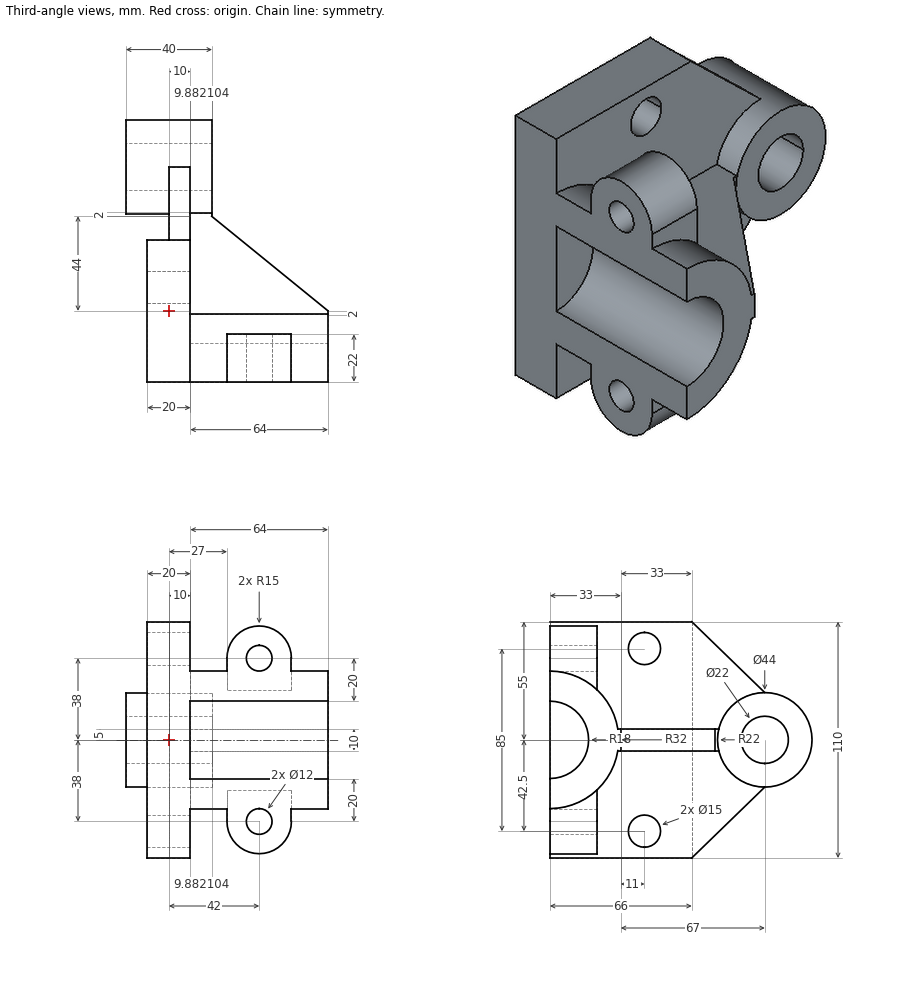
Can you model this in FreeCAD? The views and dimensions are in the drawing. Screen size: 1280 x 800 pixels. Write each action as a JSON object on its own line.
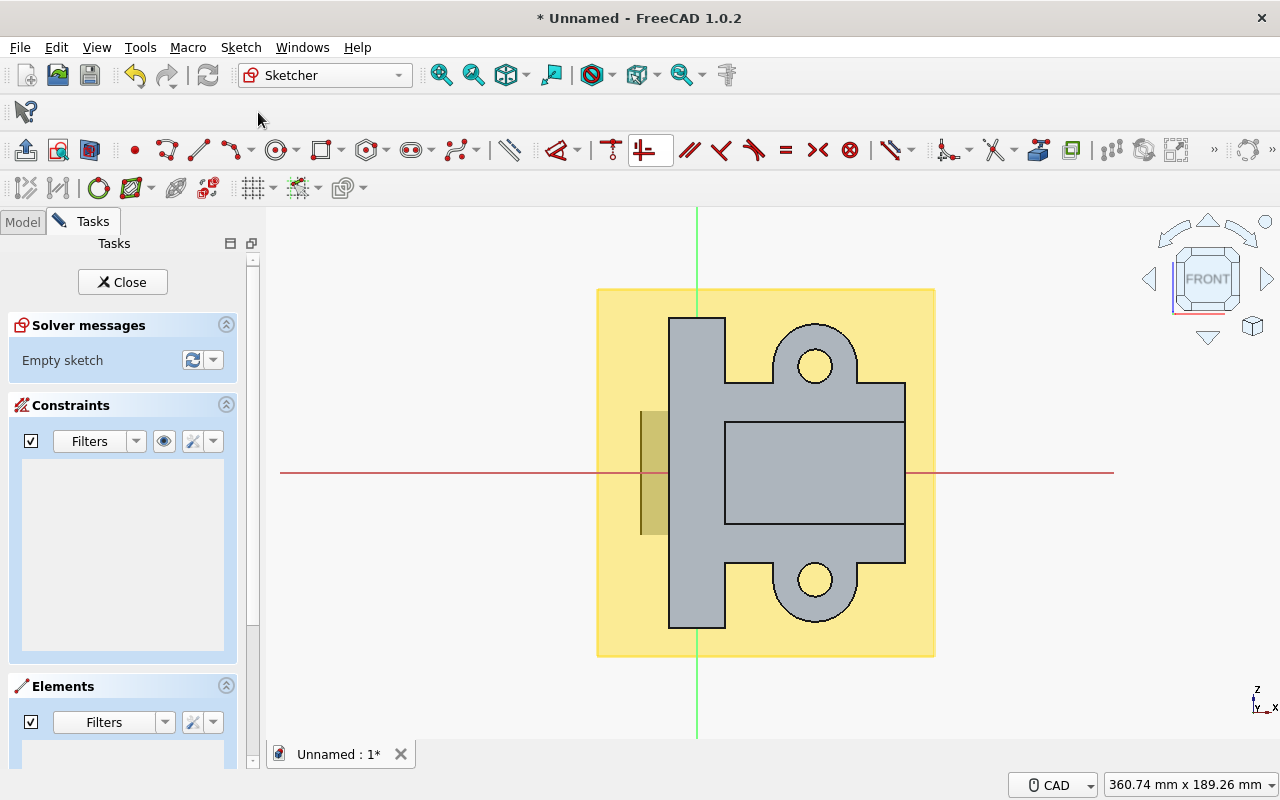
{"action": "left_click", "coordinate": [90, 150]}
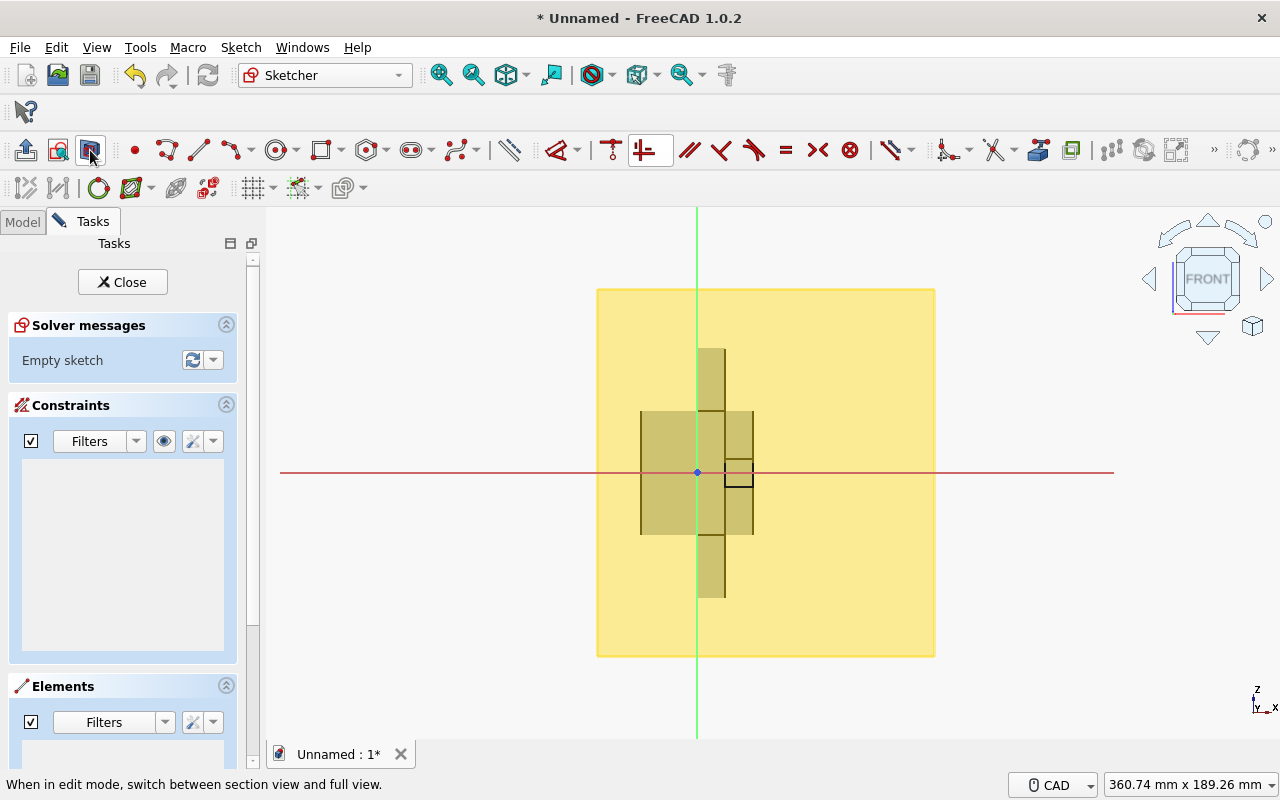
{"action": "scroll", "coordinate": [727, 473], "scroll_direction": "up", "scroll_amount": 12}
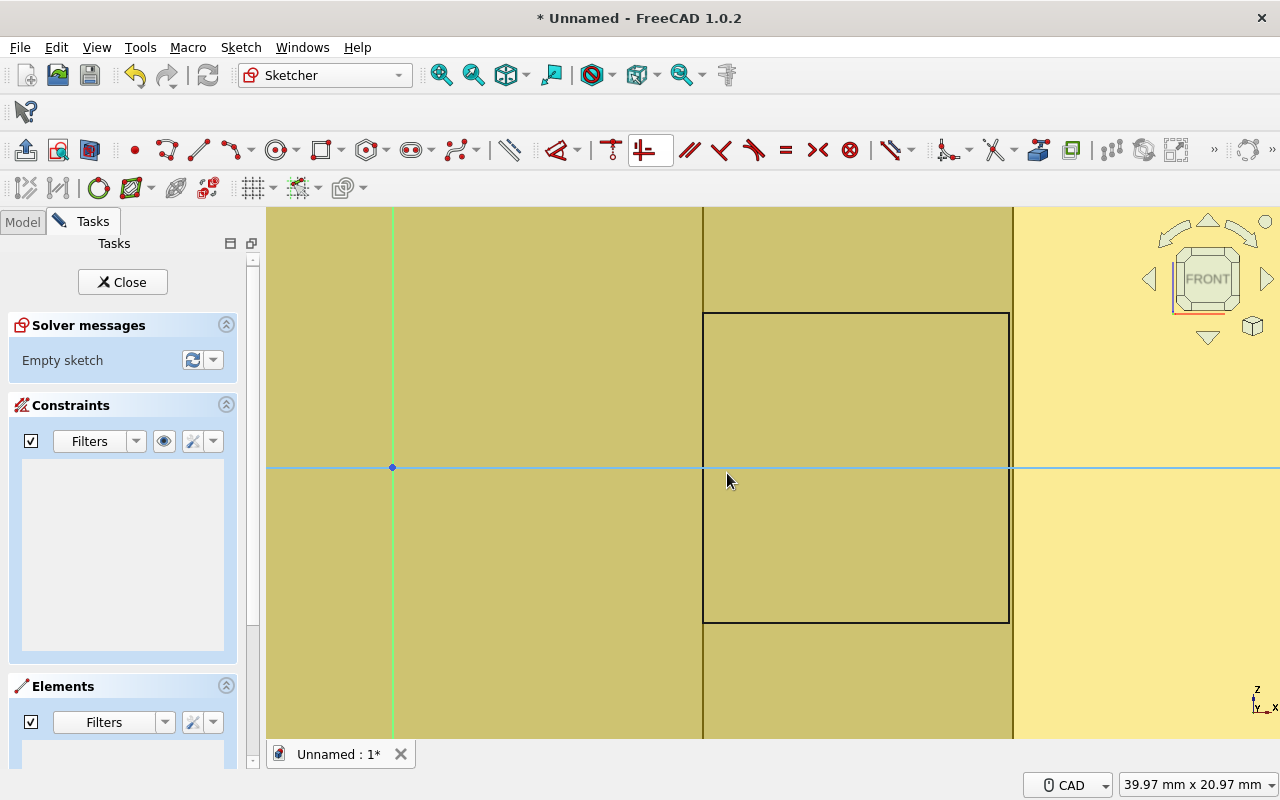
{"action": "left_click", "coordinate": [322, 150]}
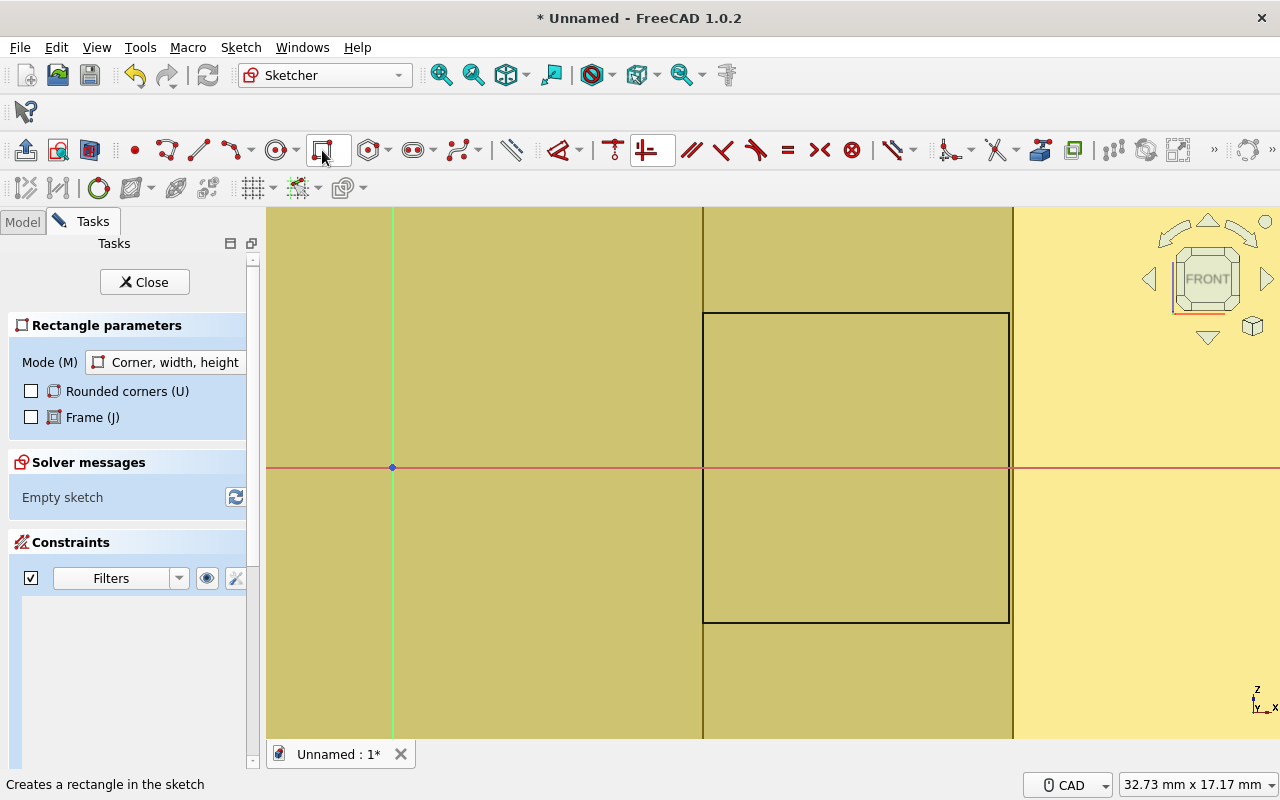
{"action": "left_click", "coordinate": [703, 313]}
{"action": "left_click", "coordinate": [1009, 623]}
{"action": "key", "text": "Escape"}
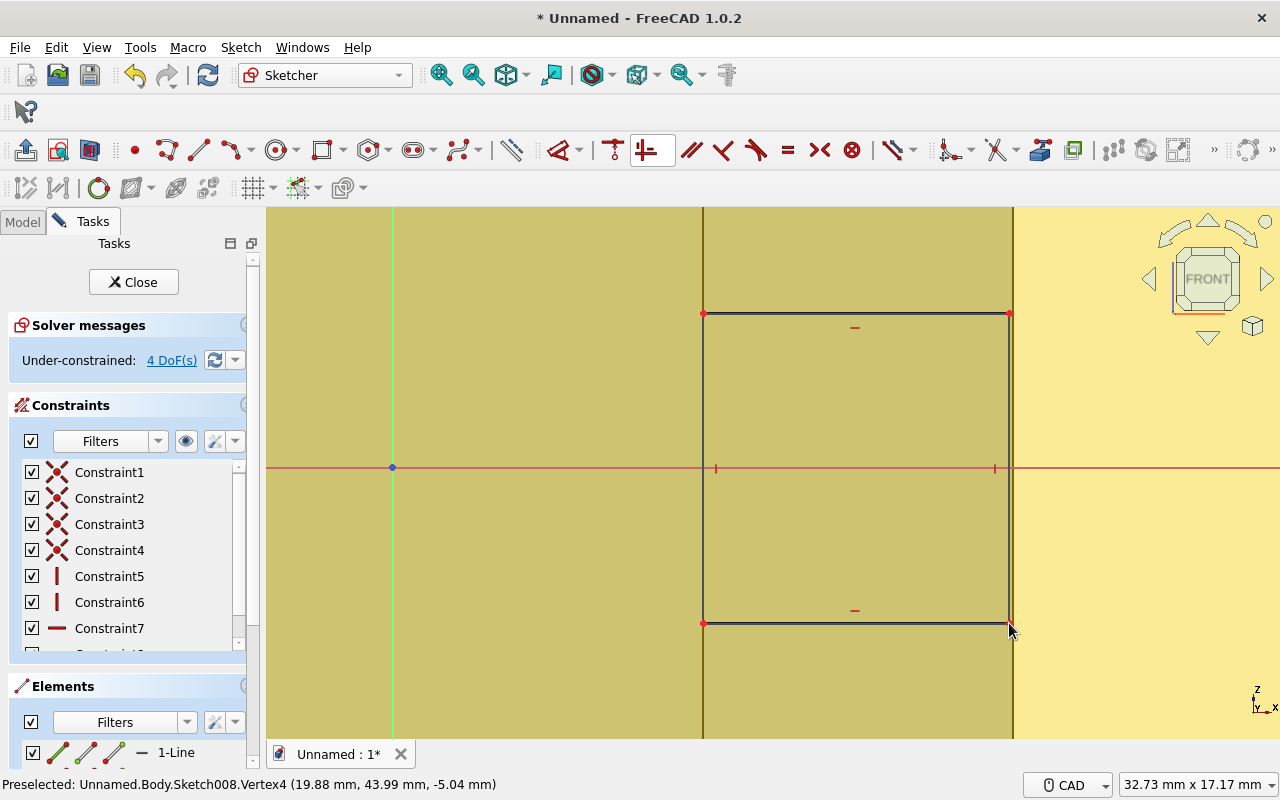
{"action": "left_click", "coordinate": [558, 150]}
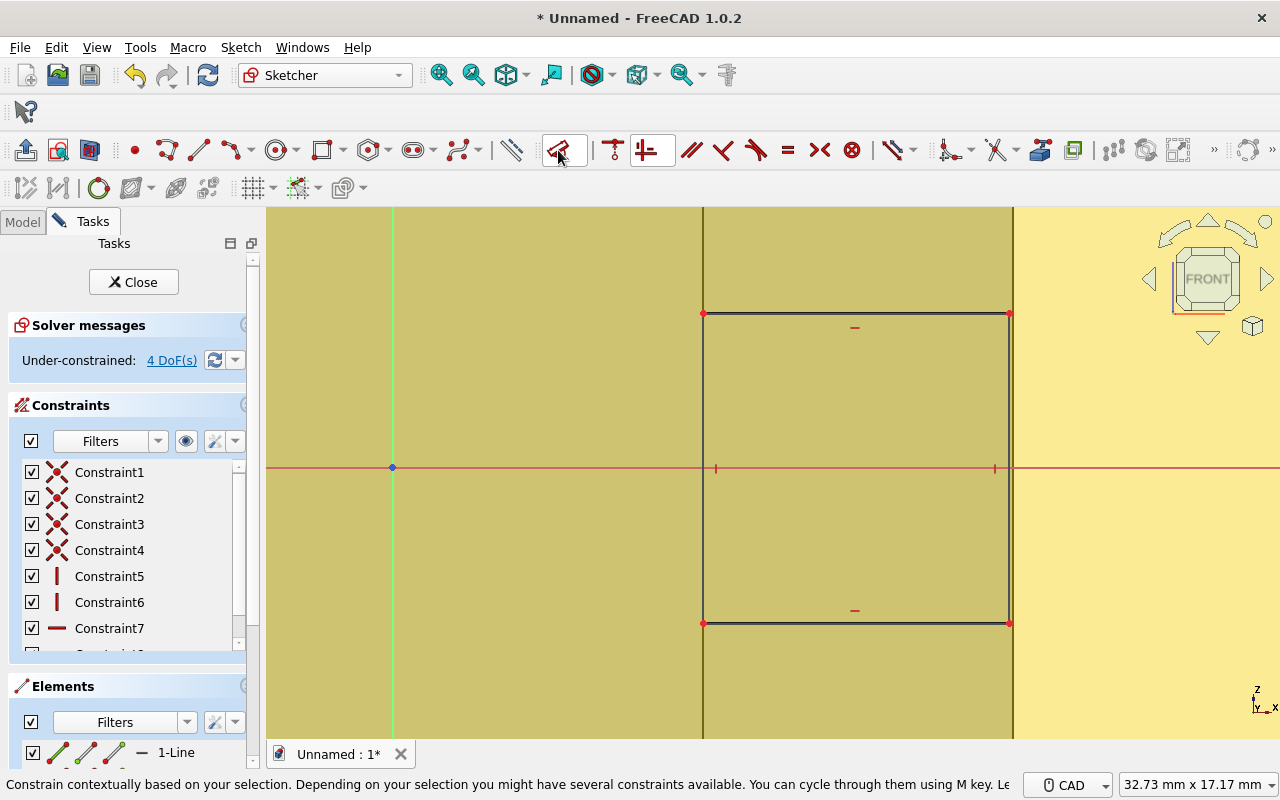
{"action": "left_click", "coordinate": [703, 407]}
{"action": "left_click", "coordinate": [737, 398]}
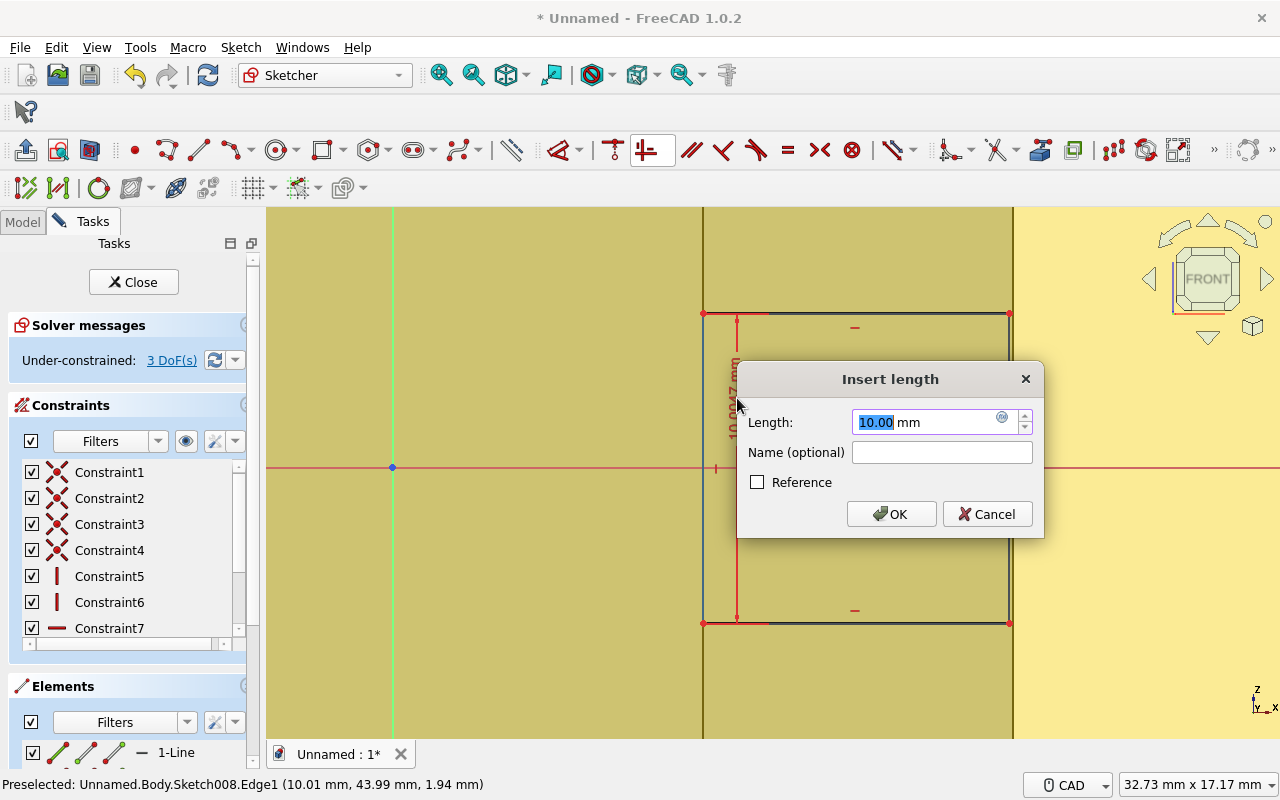
{"action": "type", "text": "10"}
{"action": "key", "text": "Return"}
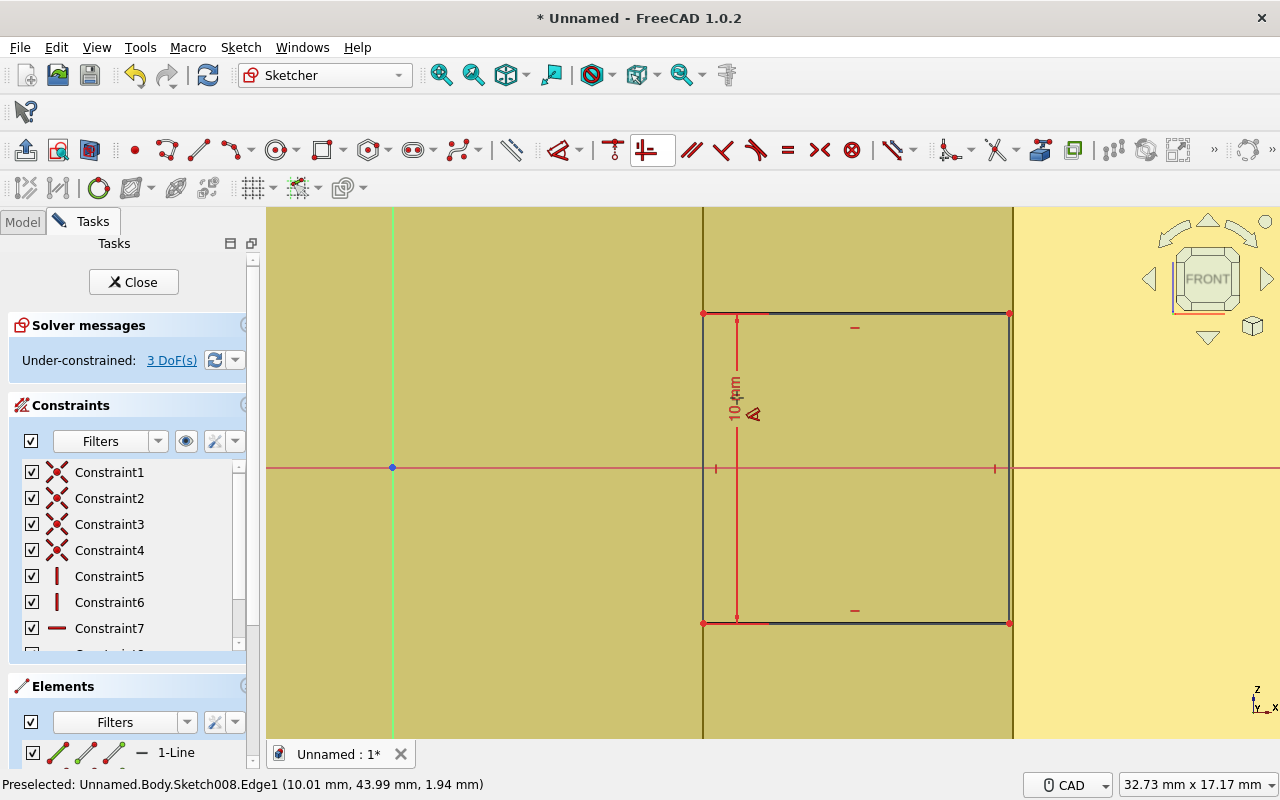
{"action": "left_click", "coordinate": [703, 314]}
{"action": "left_click", "coordinate": [359, 391]}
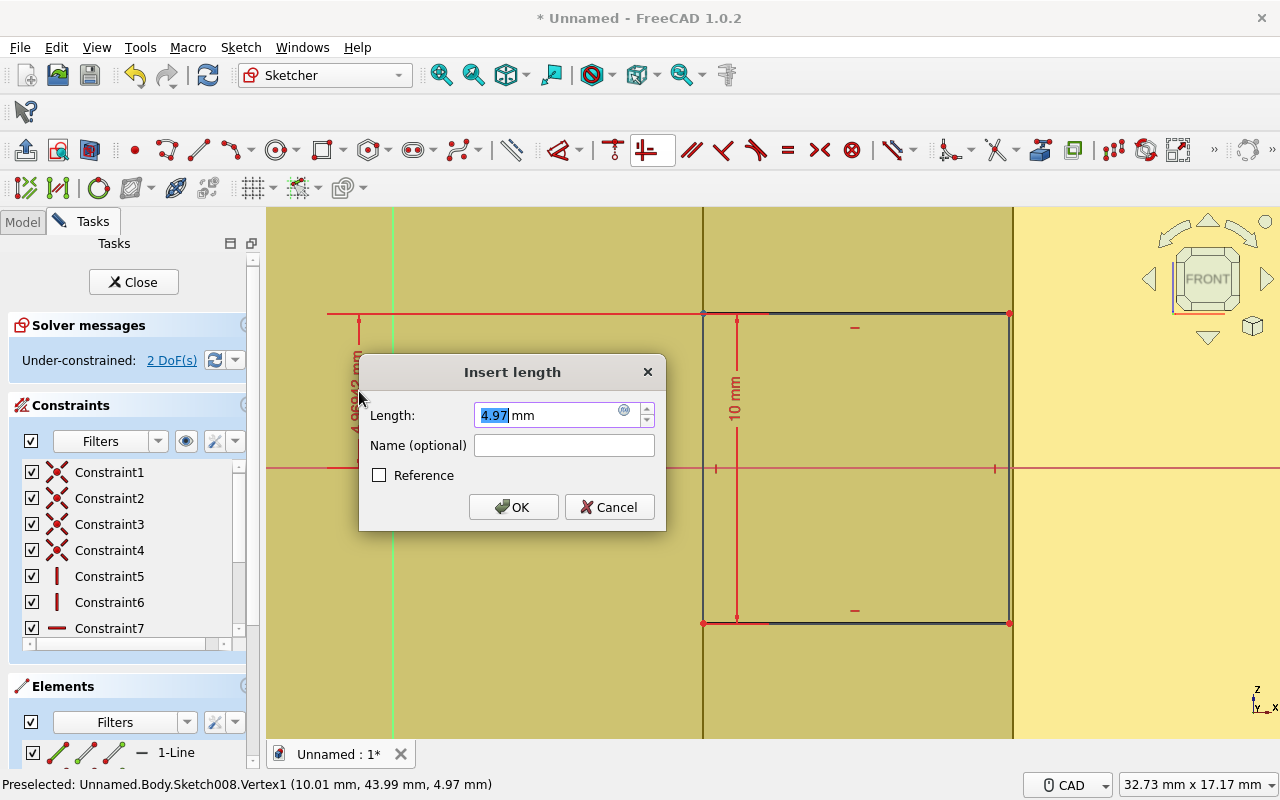
{"action": "type", "text": "5"}
{"action": "key", "text": "Return"}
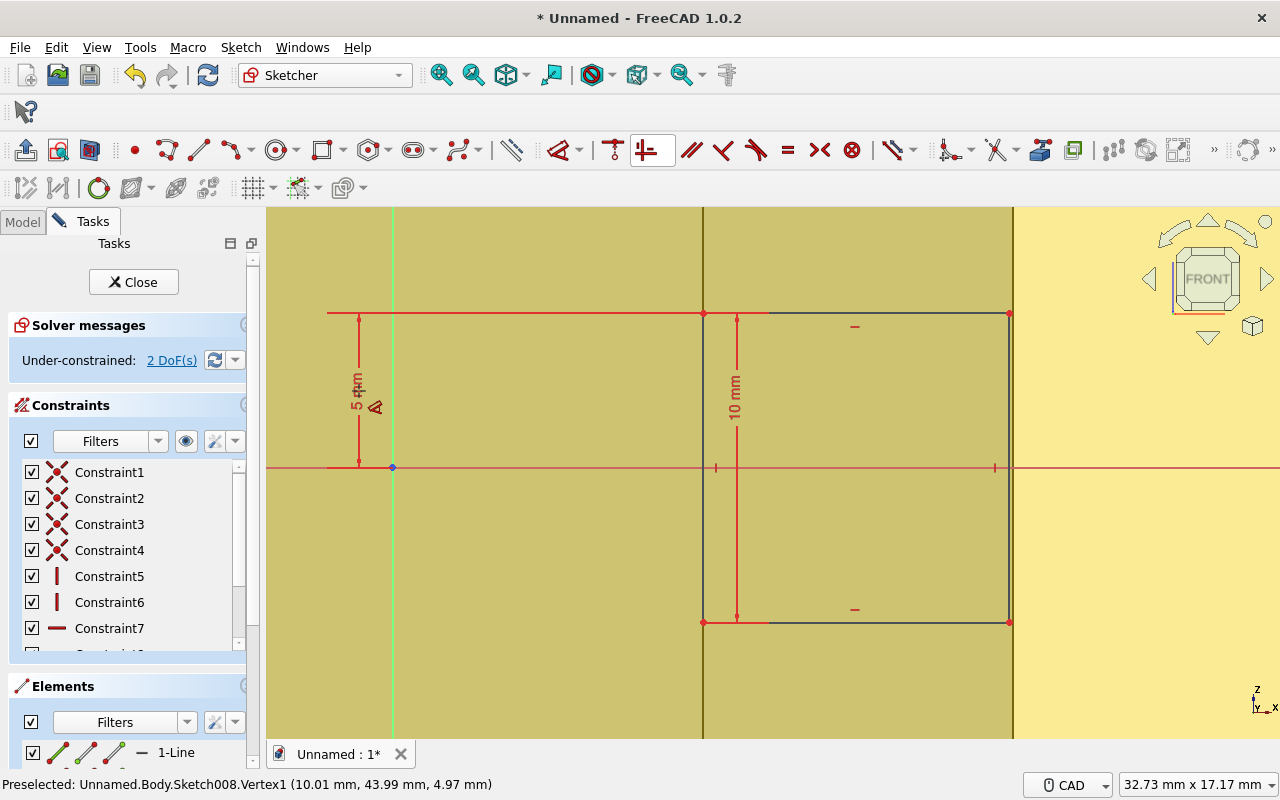
{"action": "left_click", "coordinate": [703, 313]}
{"action": "left_click", "coordinate": [548, 279]}